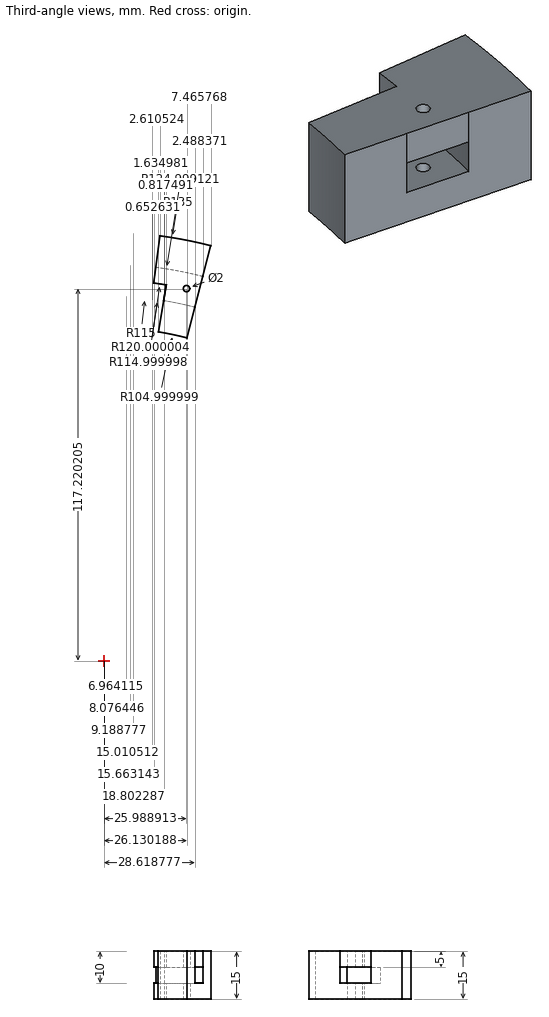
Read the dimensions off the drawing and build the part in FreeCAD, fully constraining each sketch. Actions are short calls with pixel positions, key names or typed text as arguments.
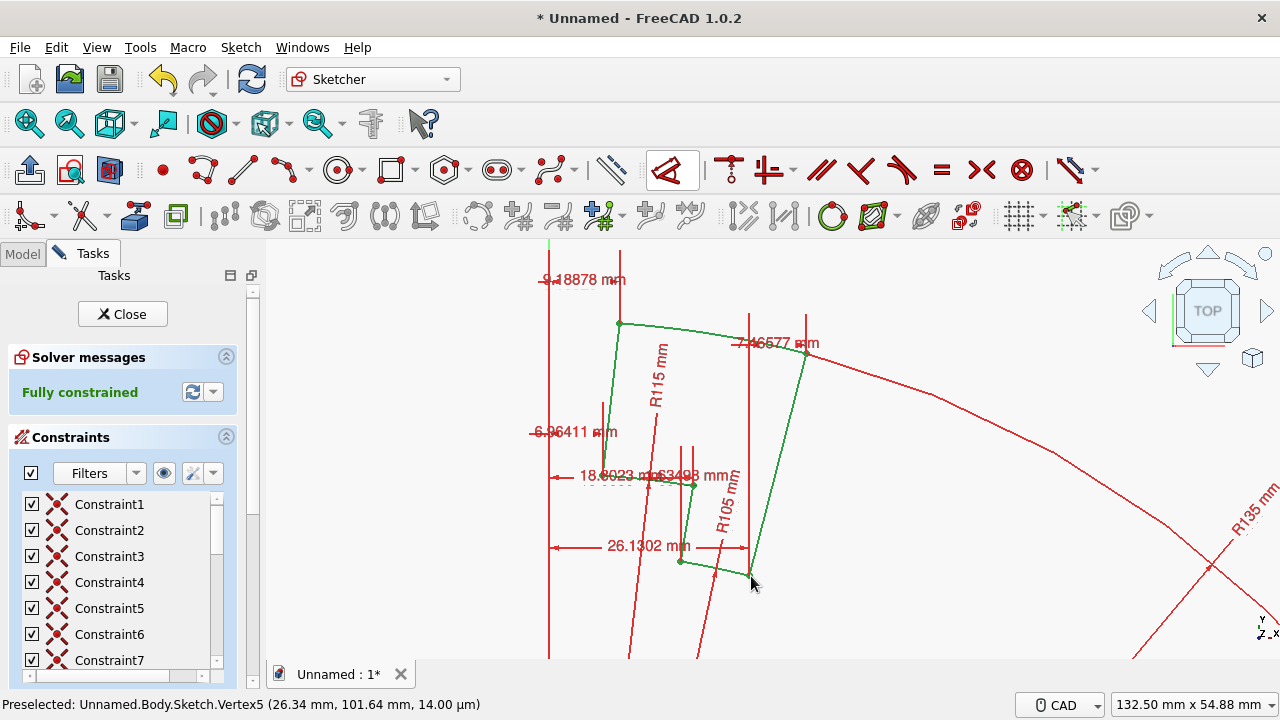
click(123, 314)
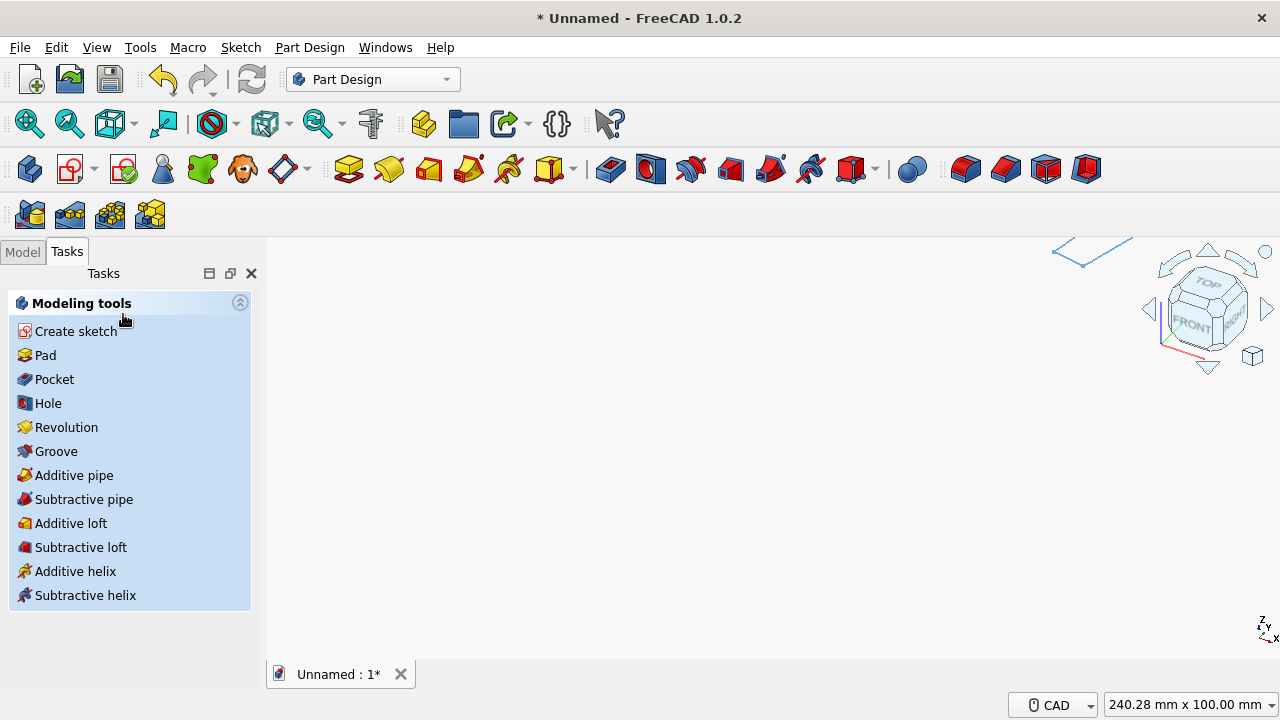
click(350, 170)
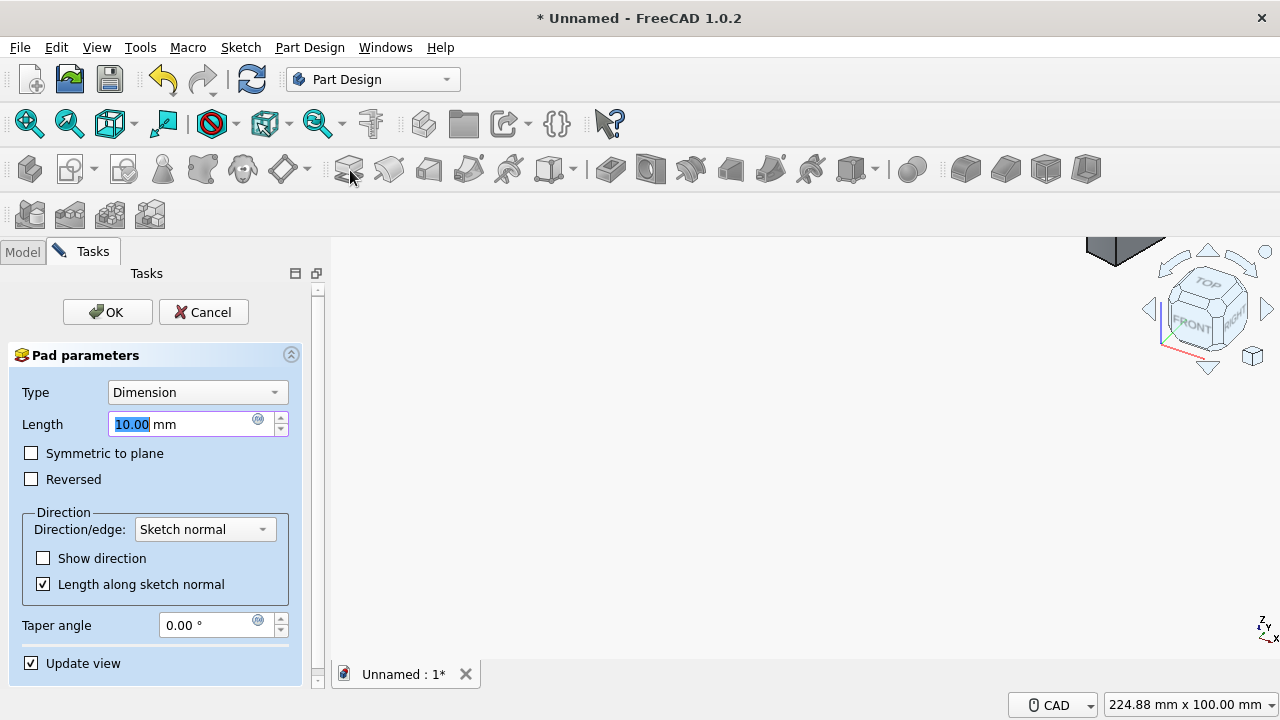
text(15)
key(Tab)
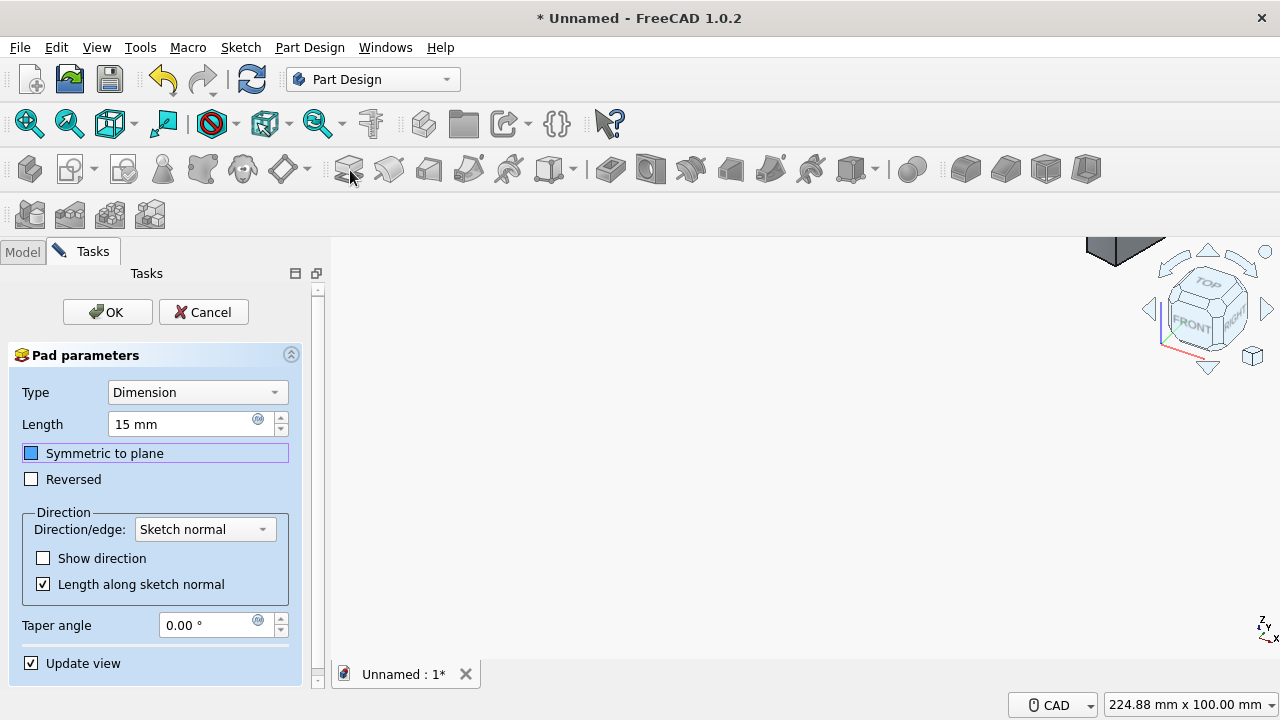
click(108, 312)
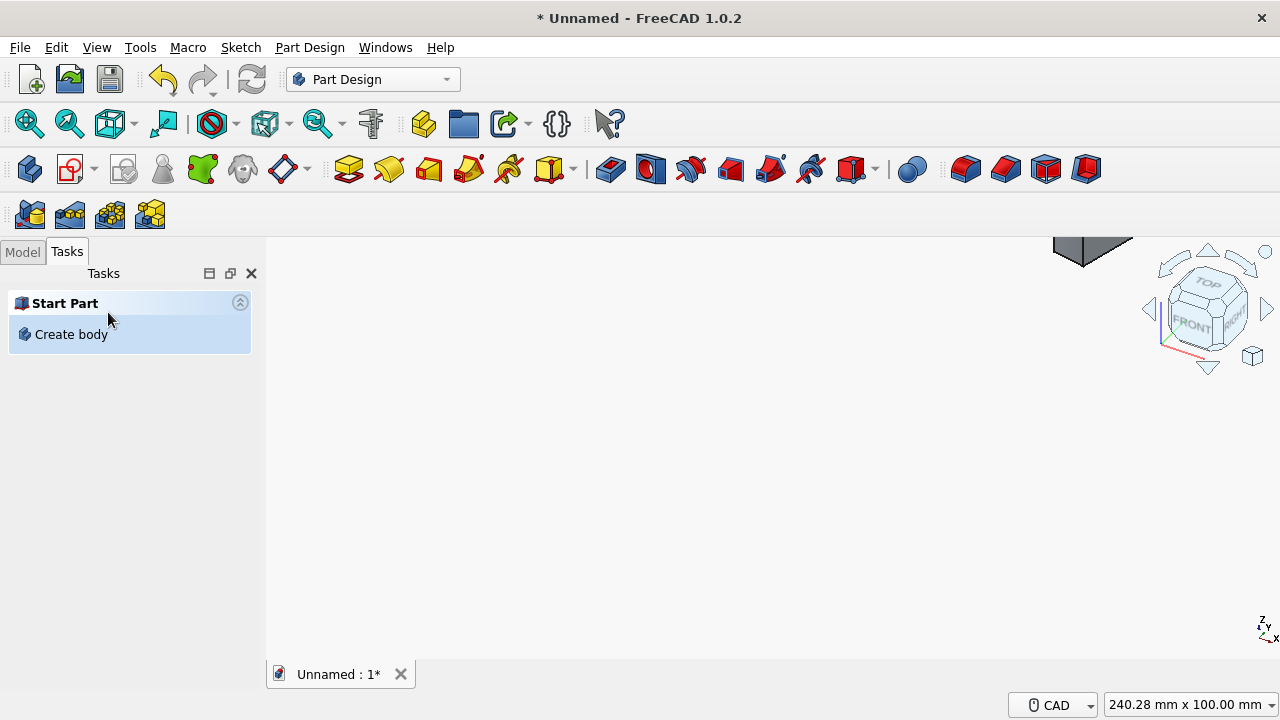
key(v)
key(f)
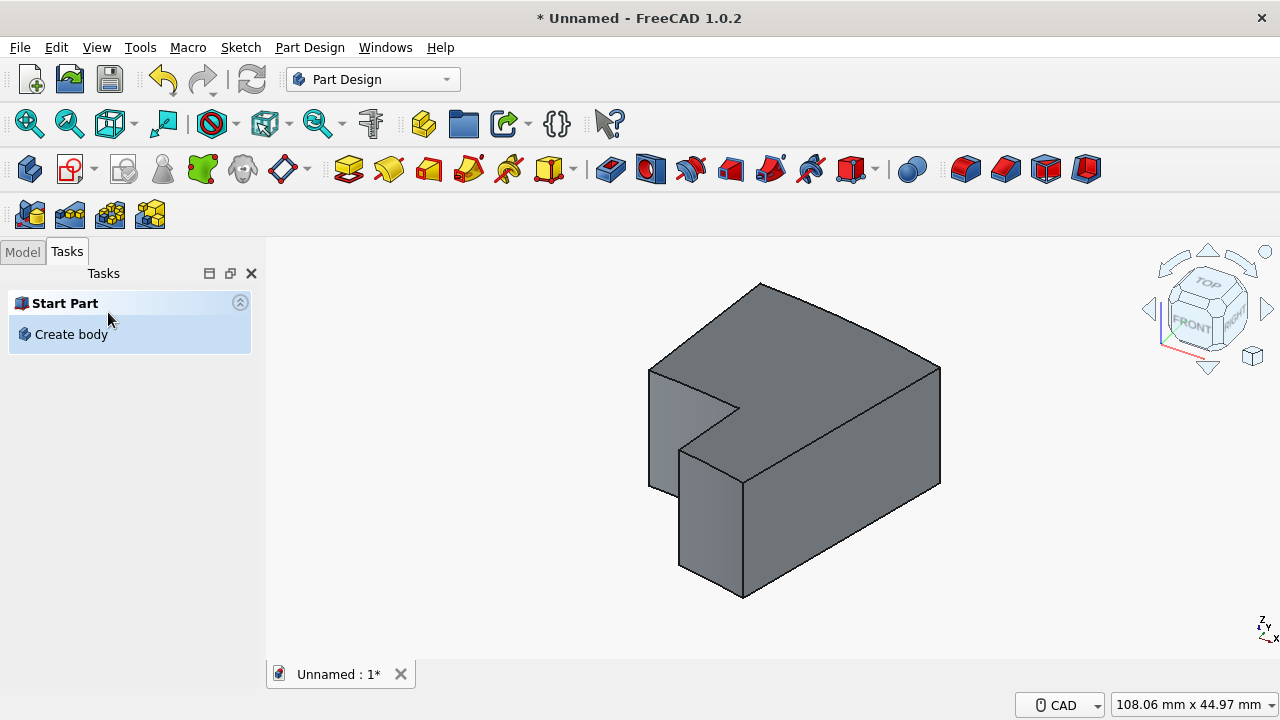
click(23, 251)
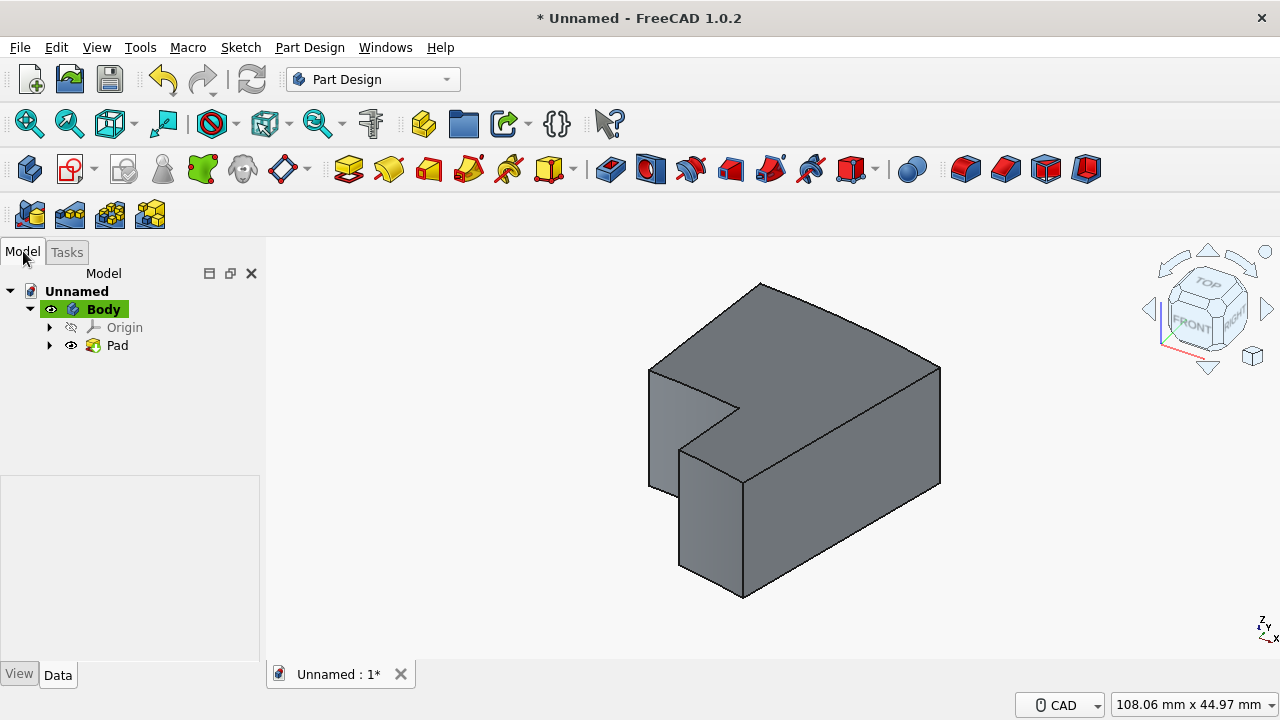
click(50, 327)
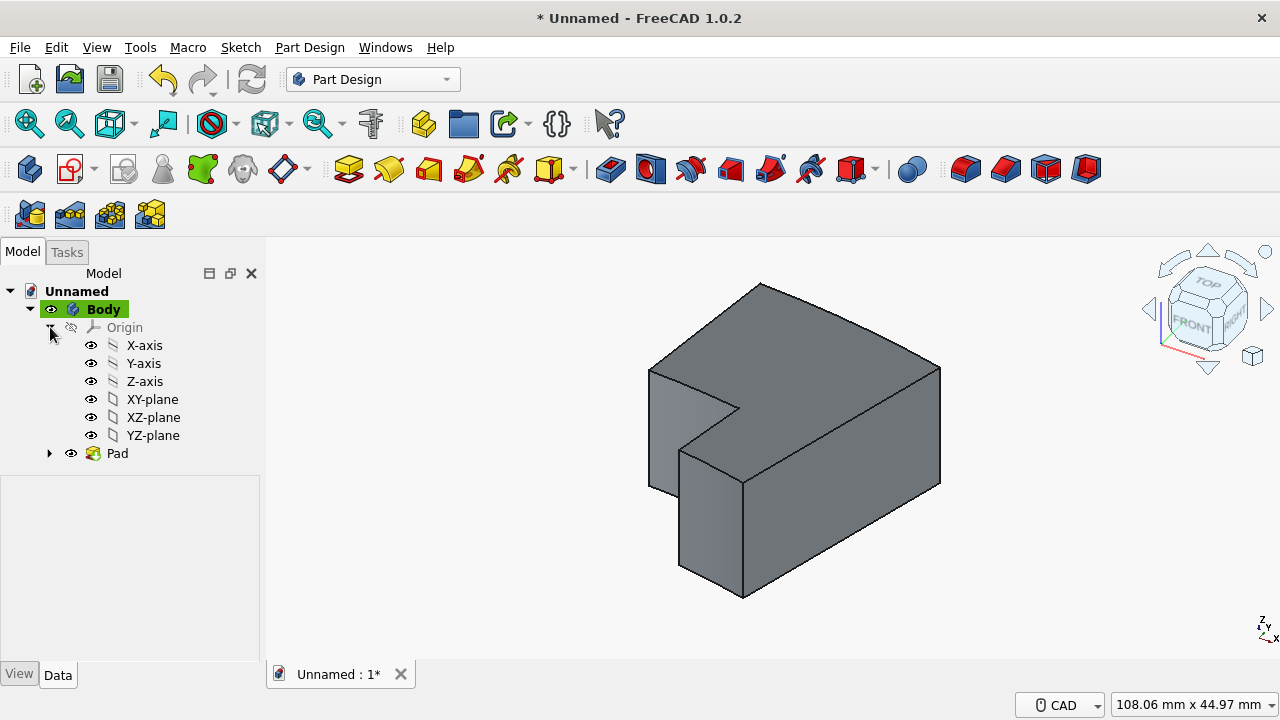
click(136, 399)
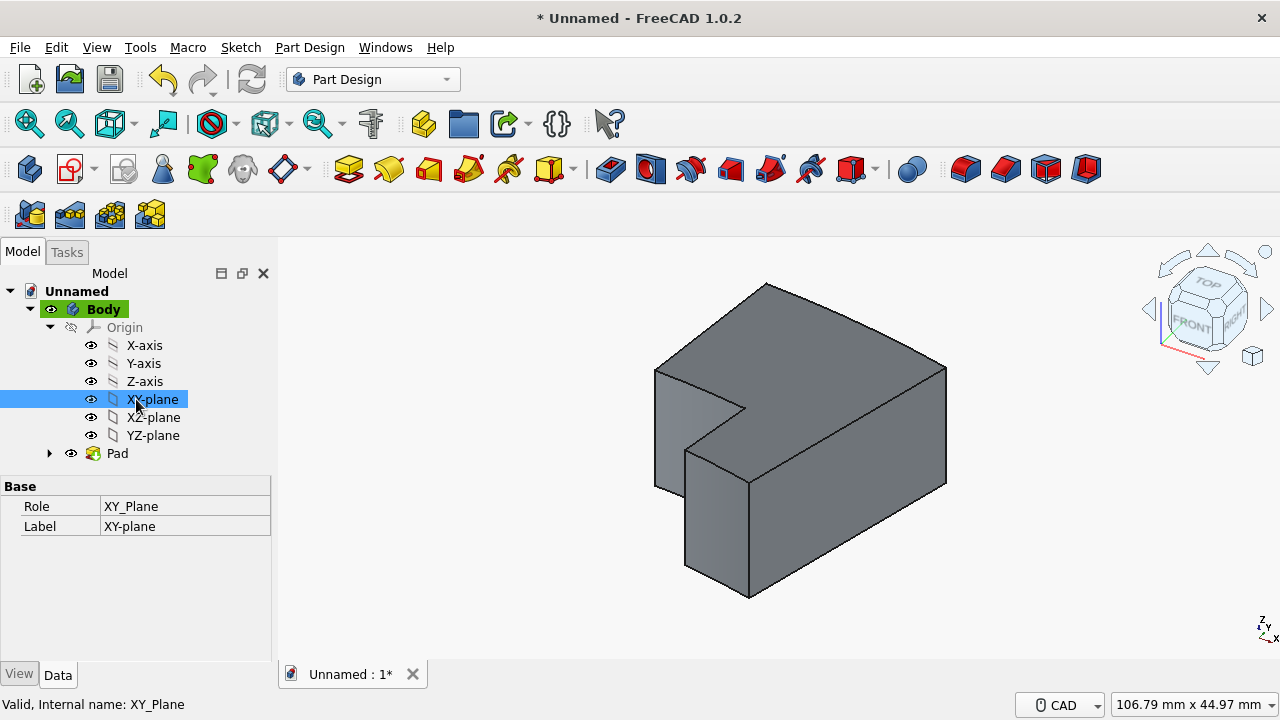
click(284, 170)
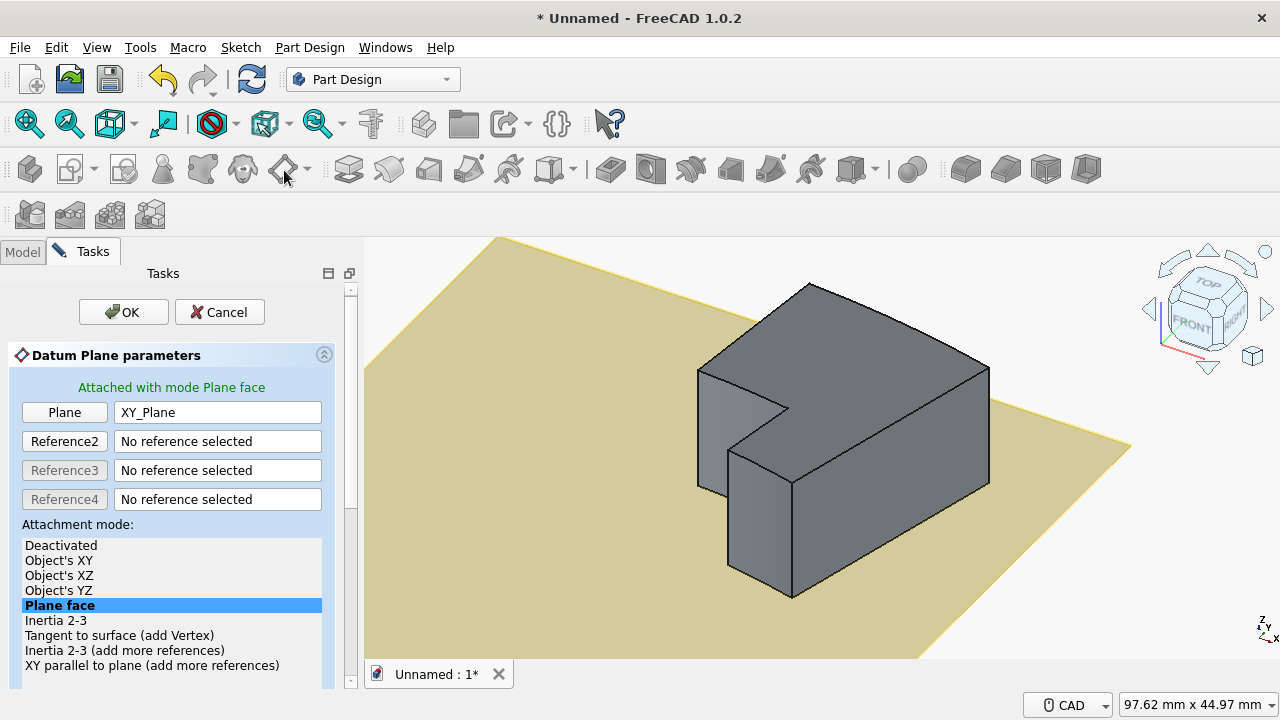
scroll(351, 486, down, 4)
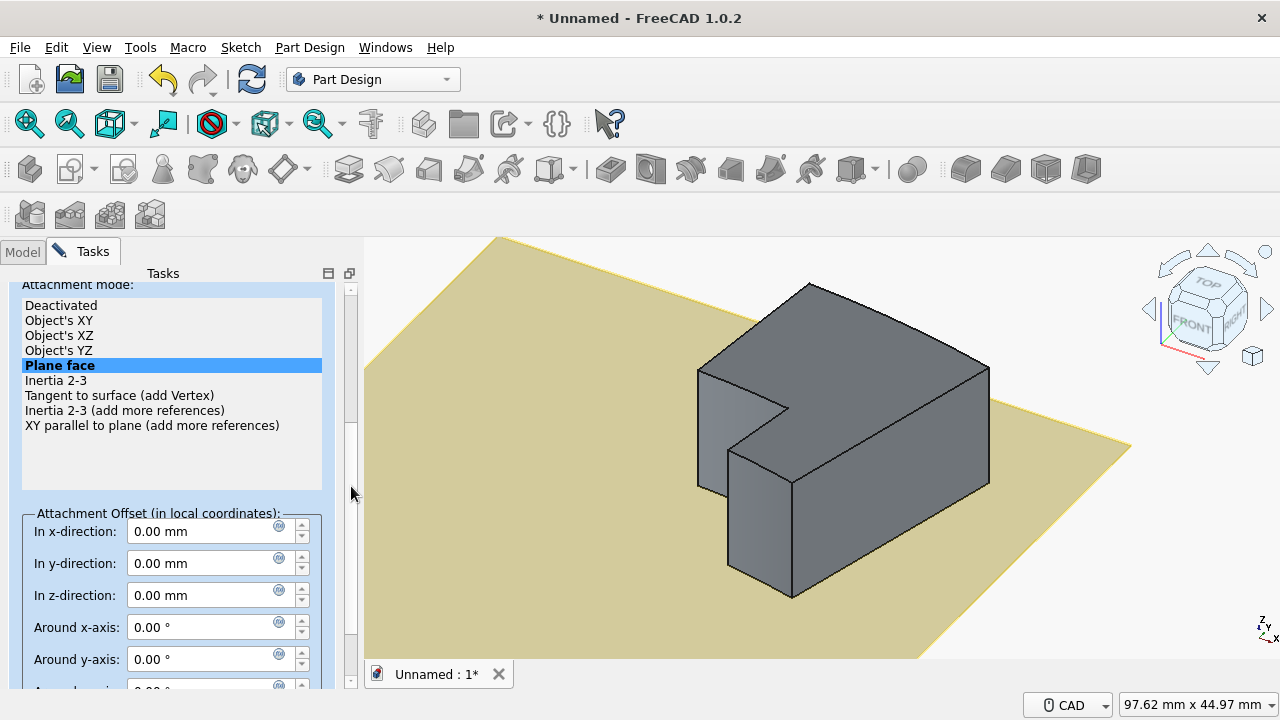
triple_click(210, 595)